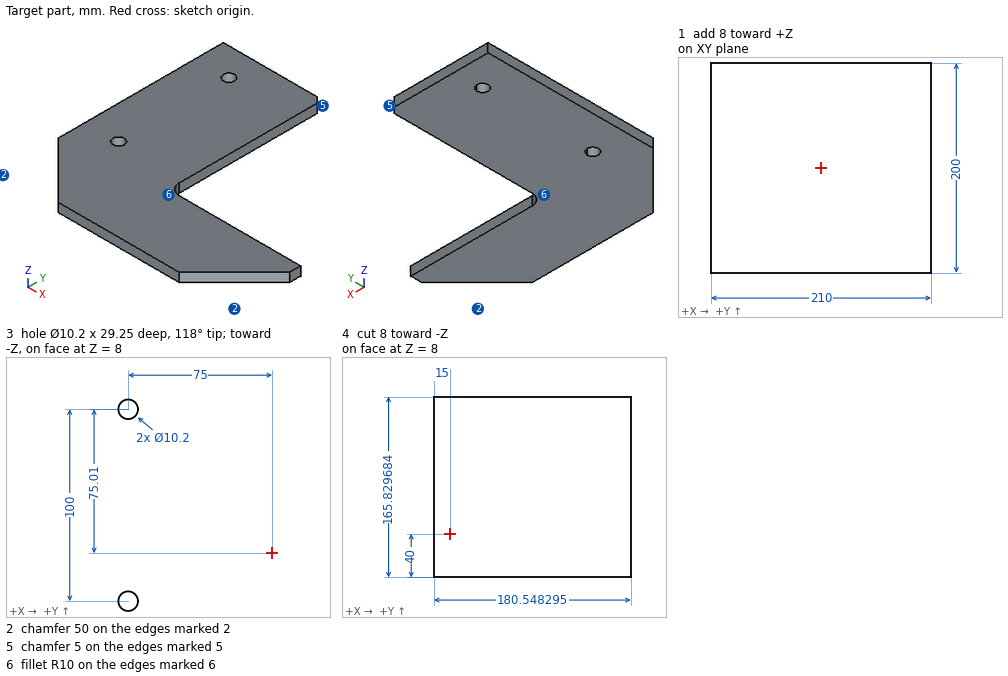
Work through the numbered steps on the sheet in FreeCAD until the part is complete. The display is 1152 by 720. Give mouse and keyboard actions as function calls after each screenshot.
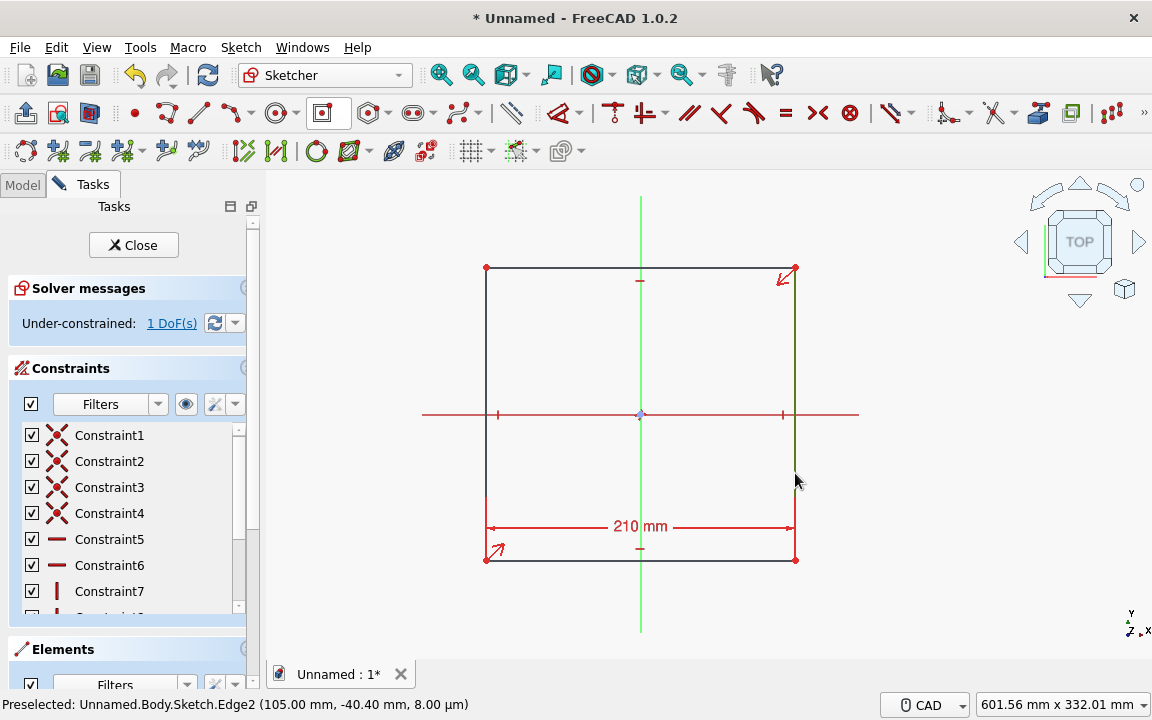
key(i)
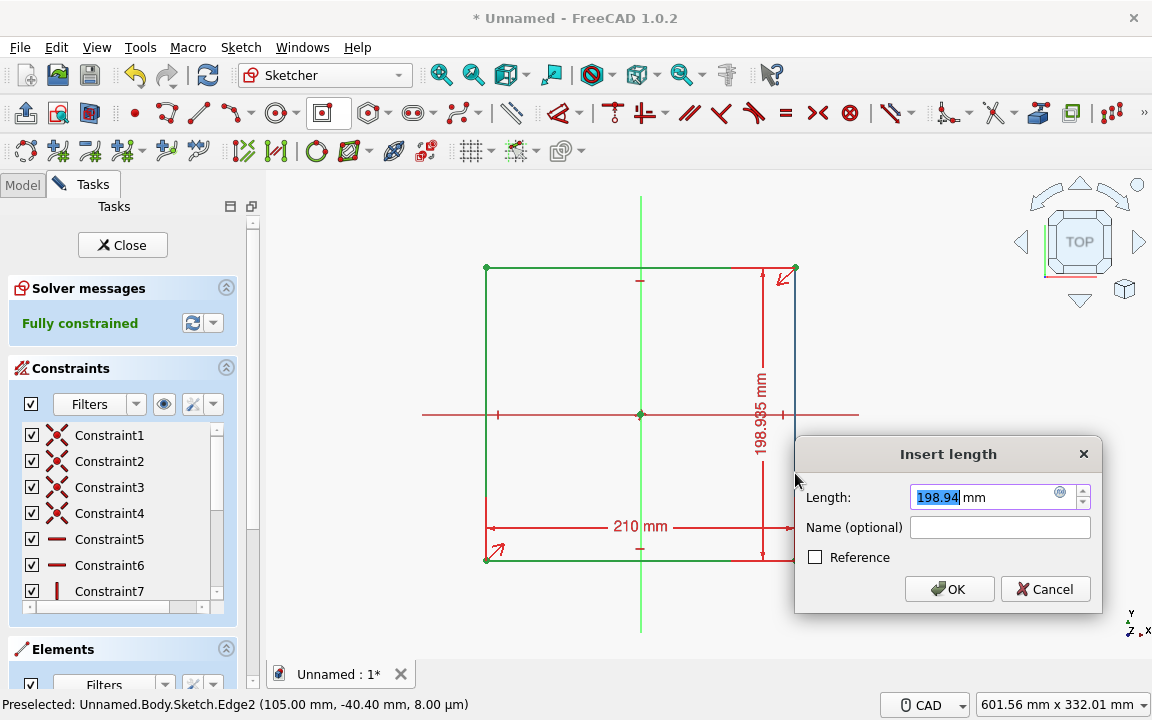
text(200)
key(Return)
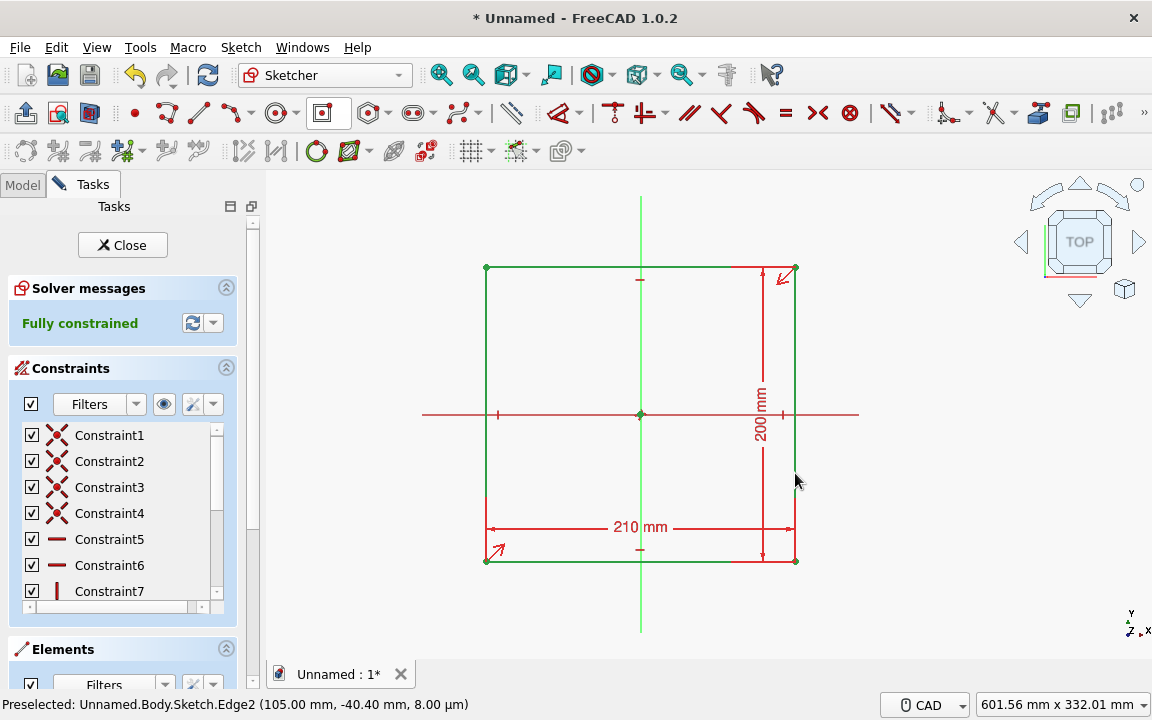
click(123, 245)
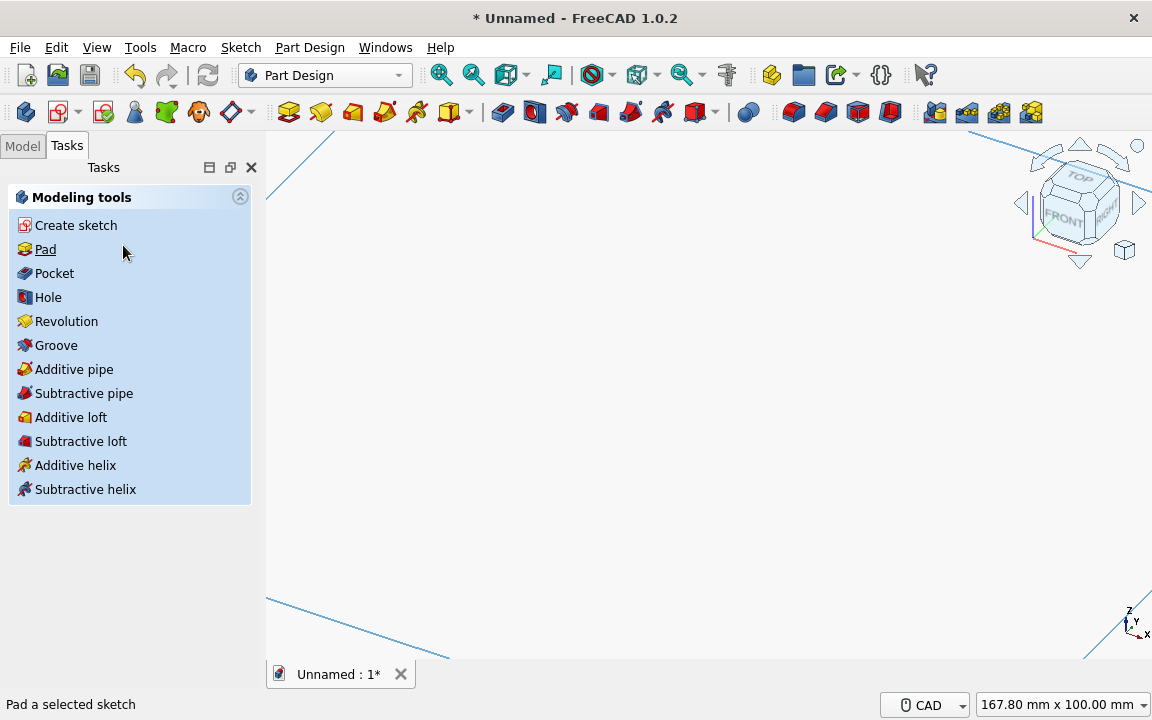
click(290, 112)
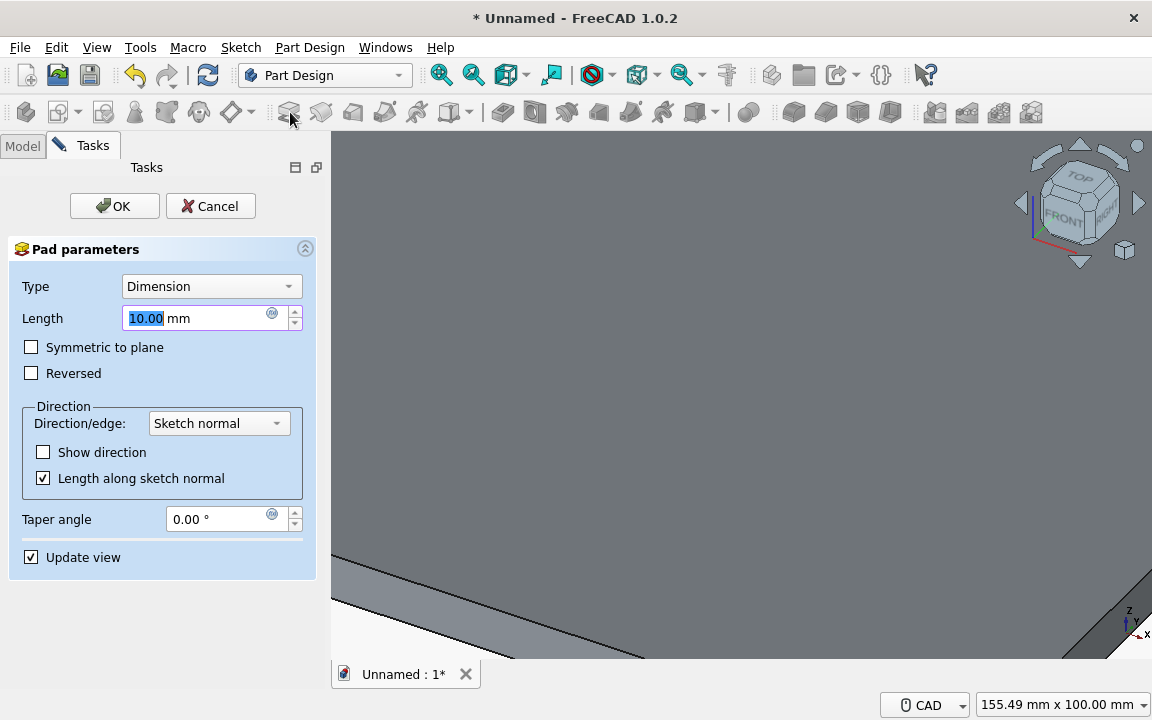
text(8)
key(Tab)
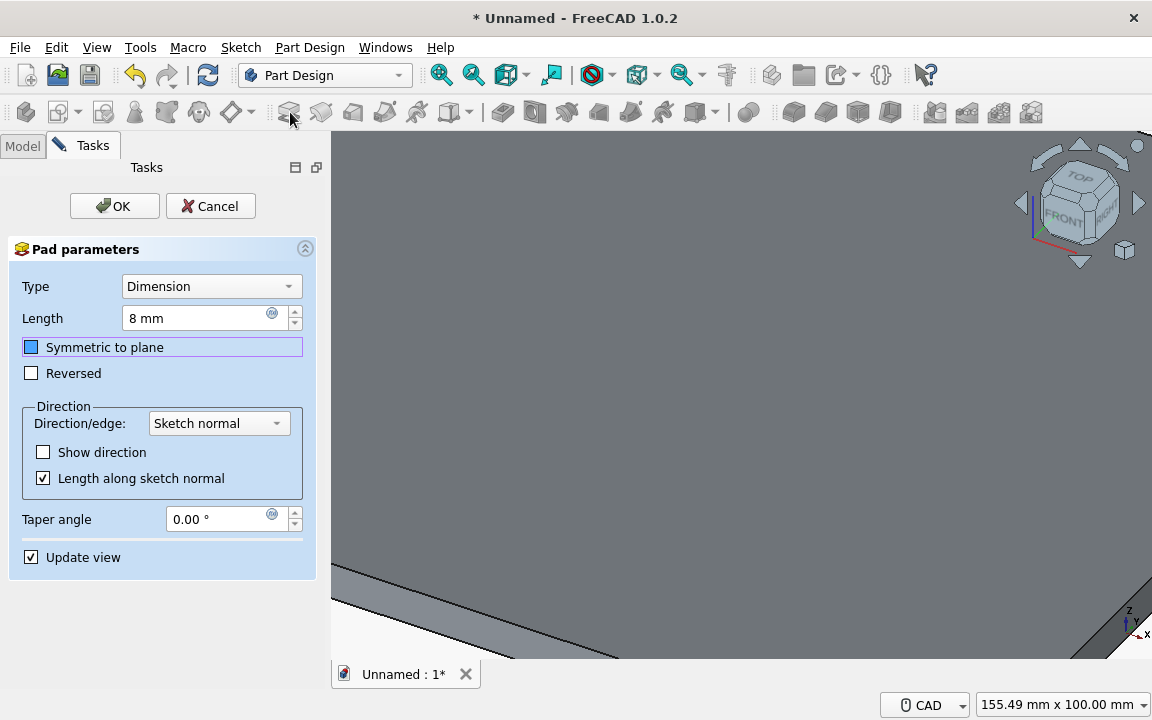
click(115, 206)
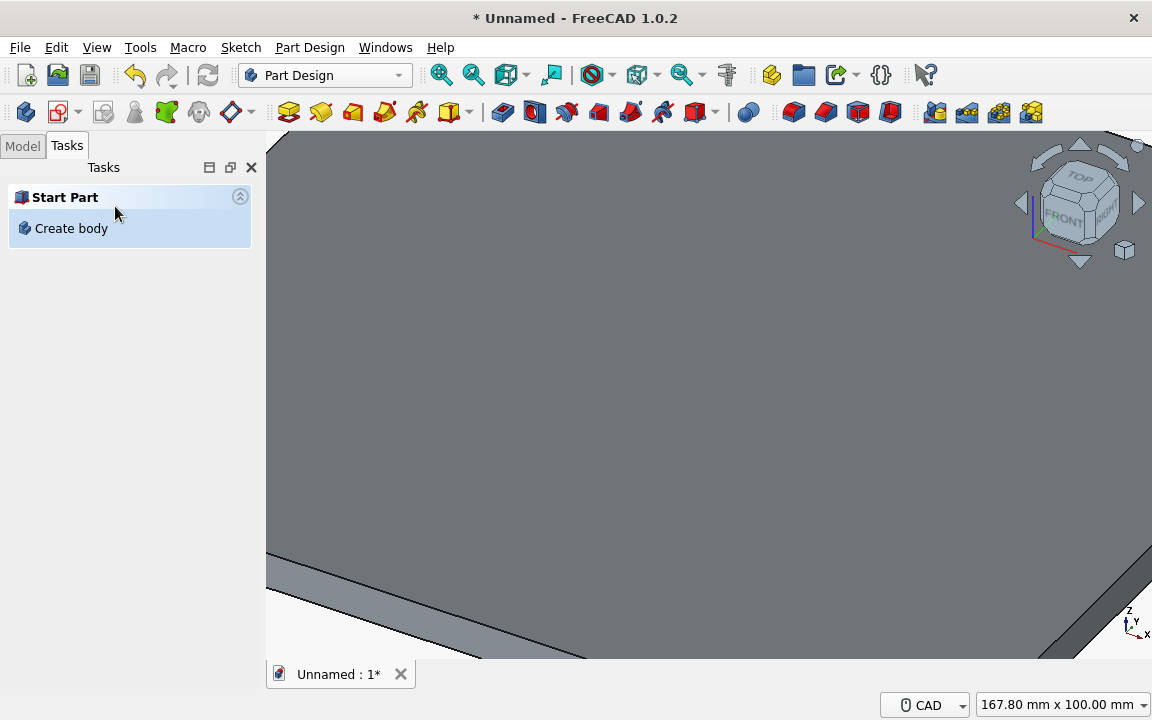
key(v)
key(f)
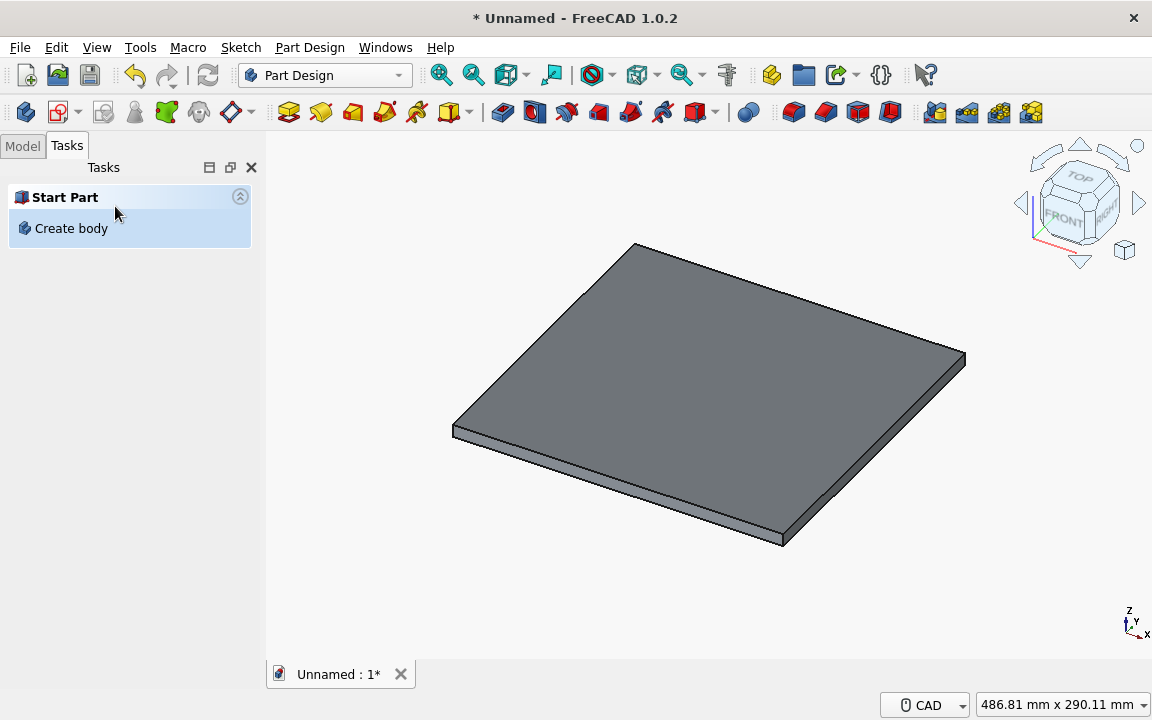
click(783, 540)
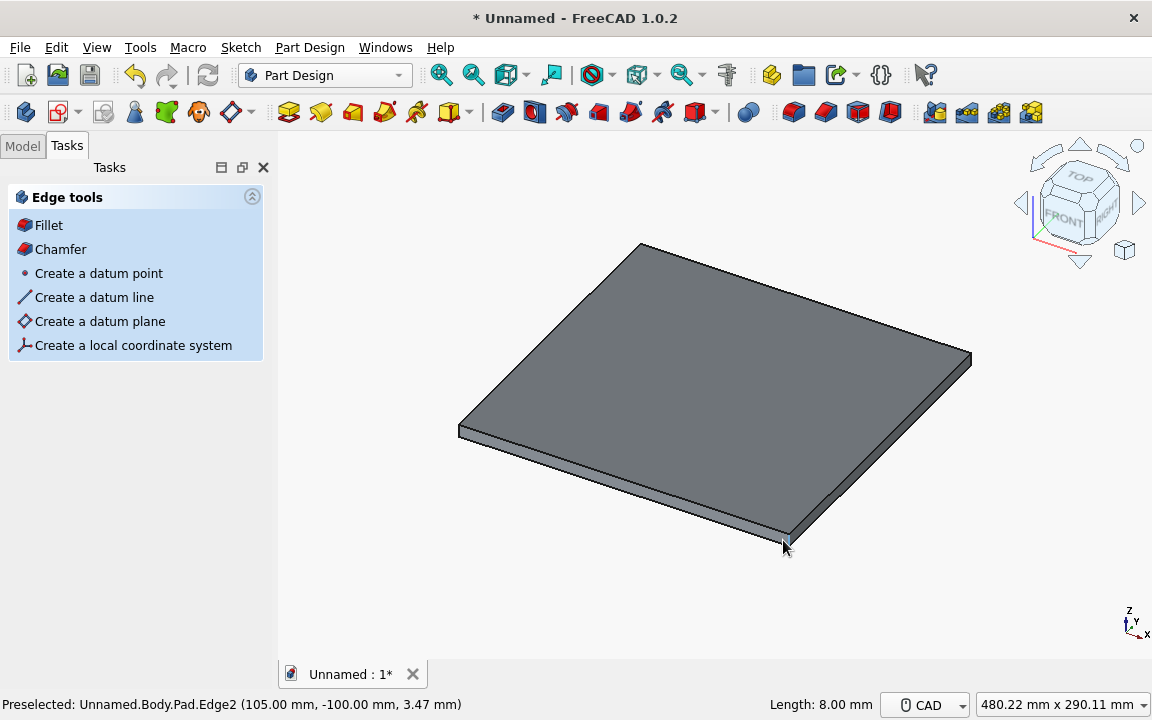
scroll(459, 430, up, 6)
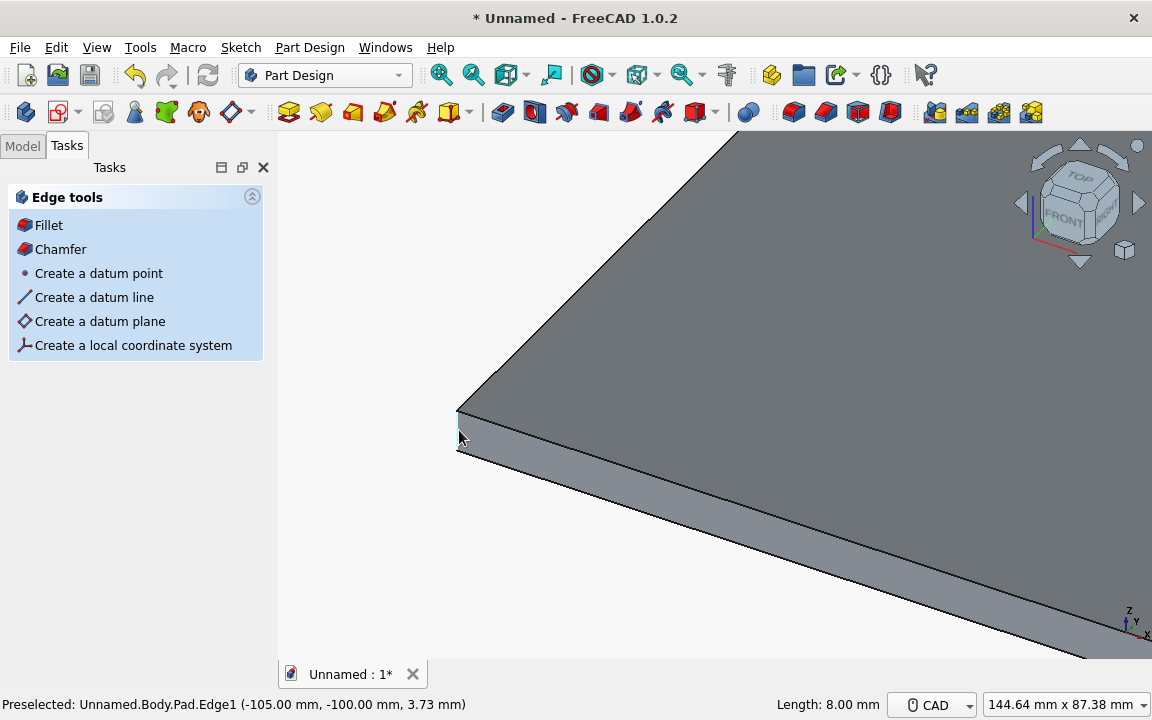
key(v)
key(f)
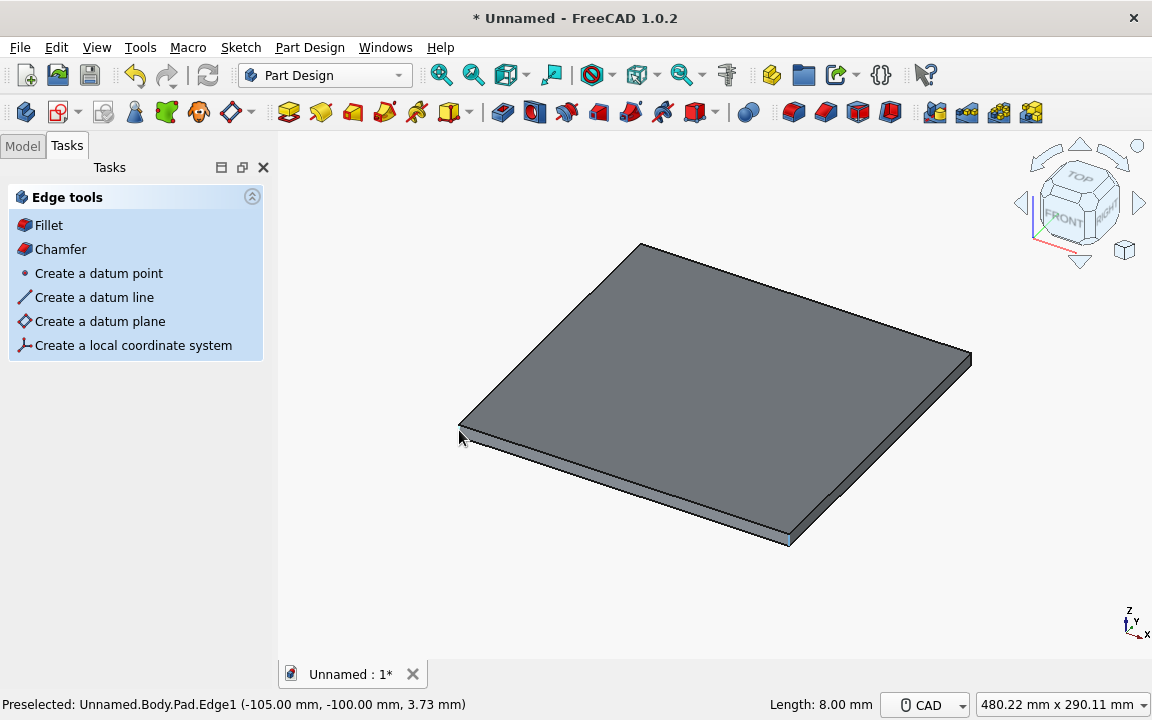
key(0)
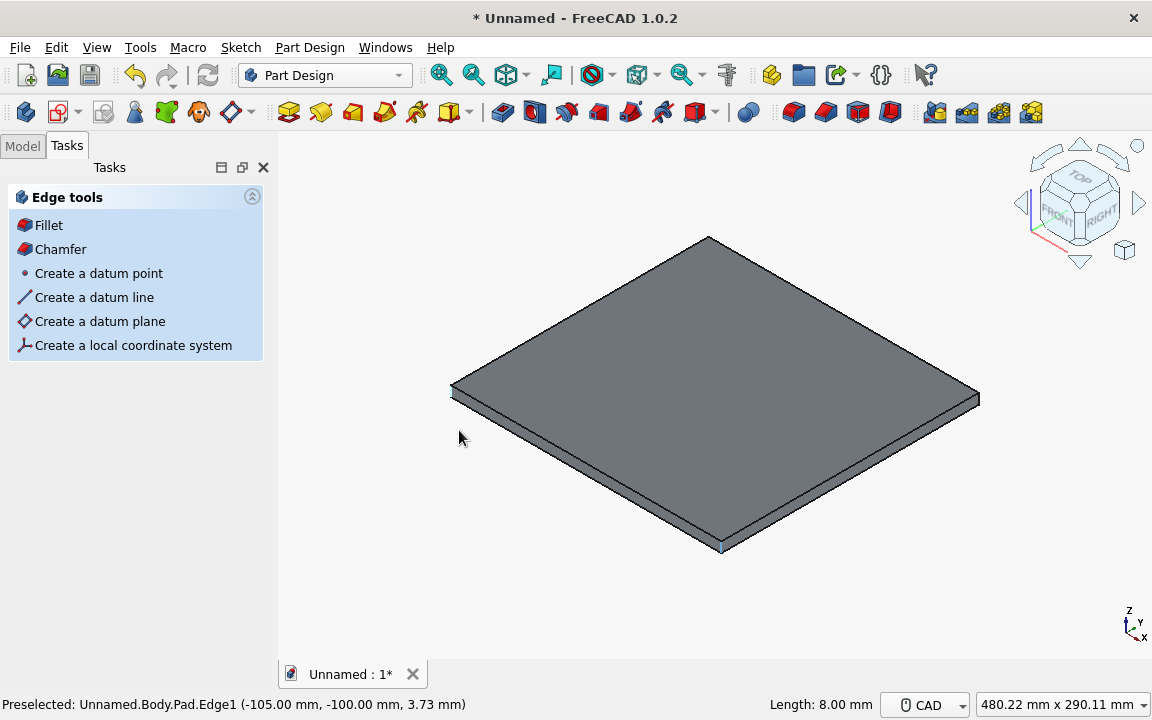
scroll(451, 390, up, 6)